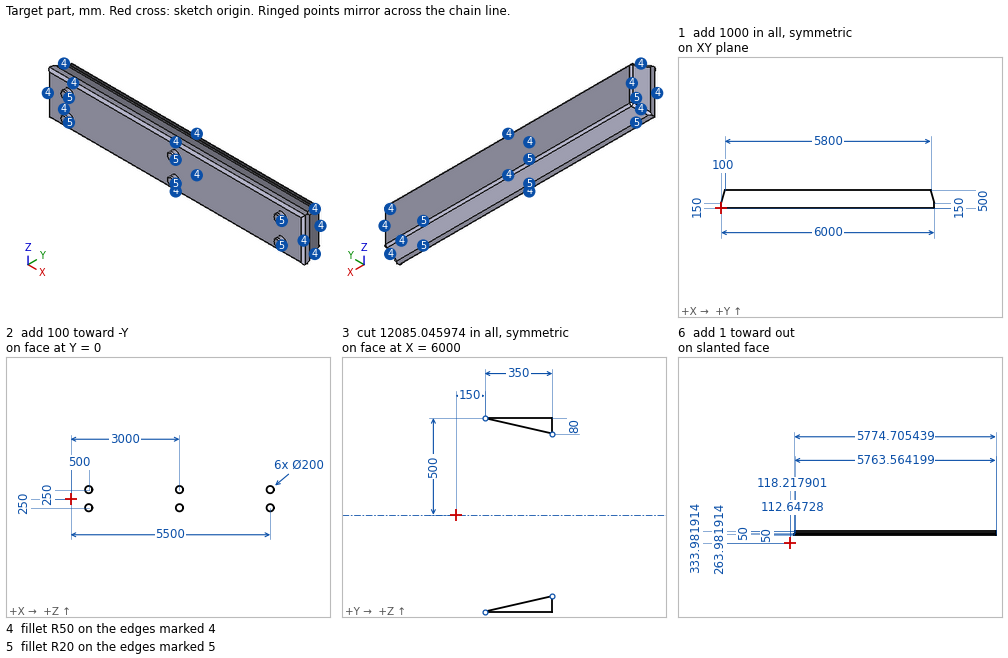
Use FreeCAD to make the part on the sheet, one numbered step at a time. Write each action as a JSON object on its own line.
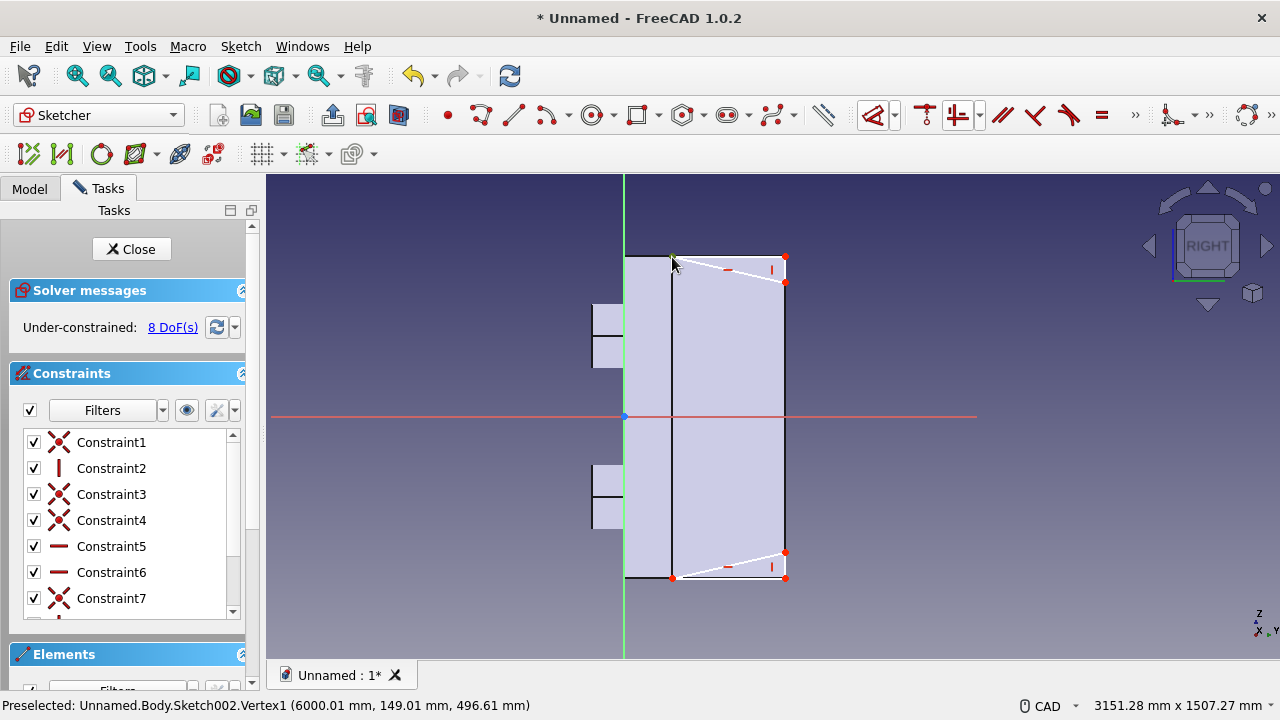
{"action": "left_click", "coordinate": [672, 579]}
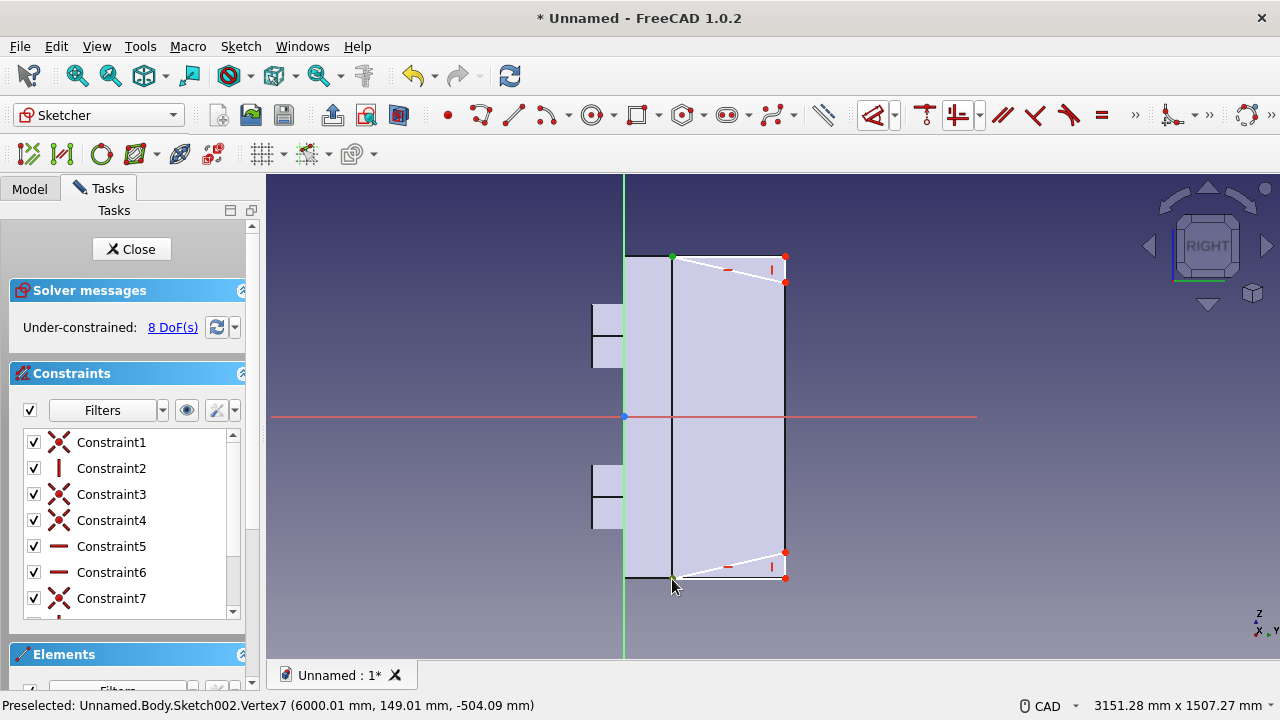
{"action": "left_click", "coordinate": [353, 417]}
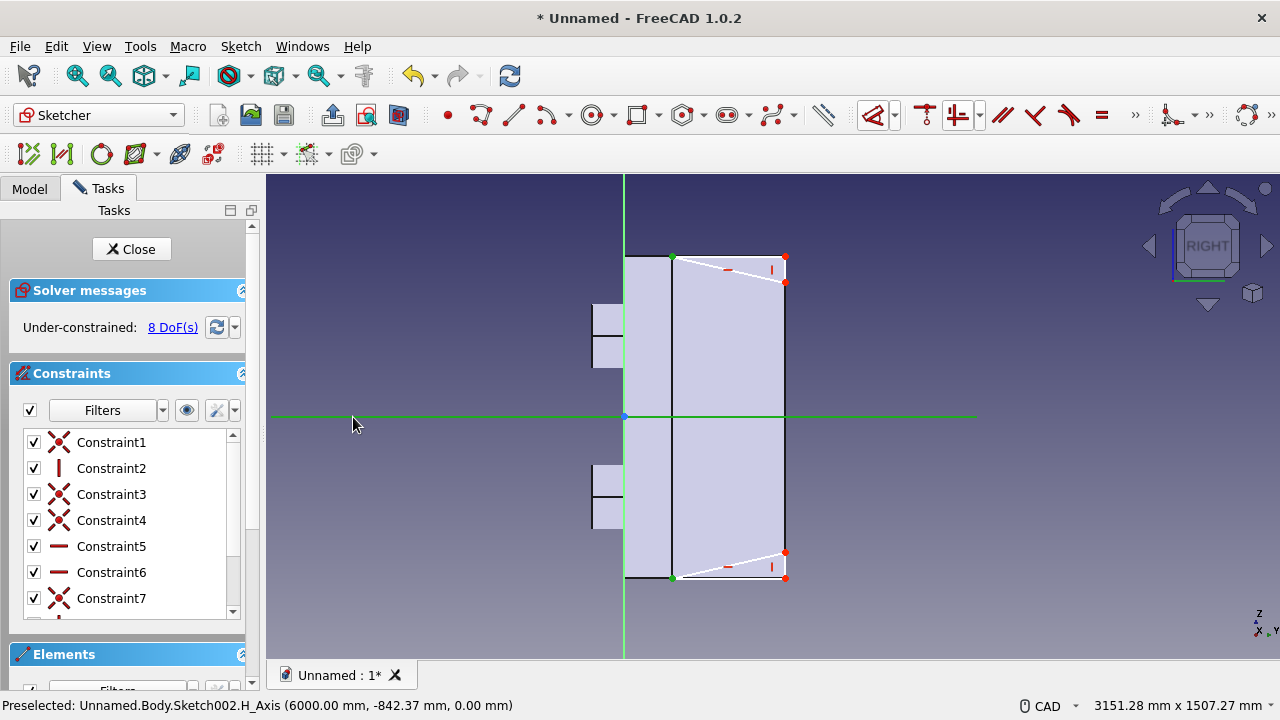
{"action": "key", "text": "s"}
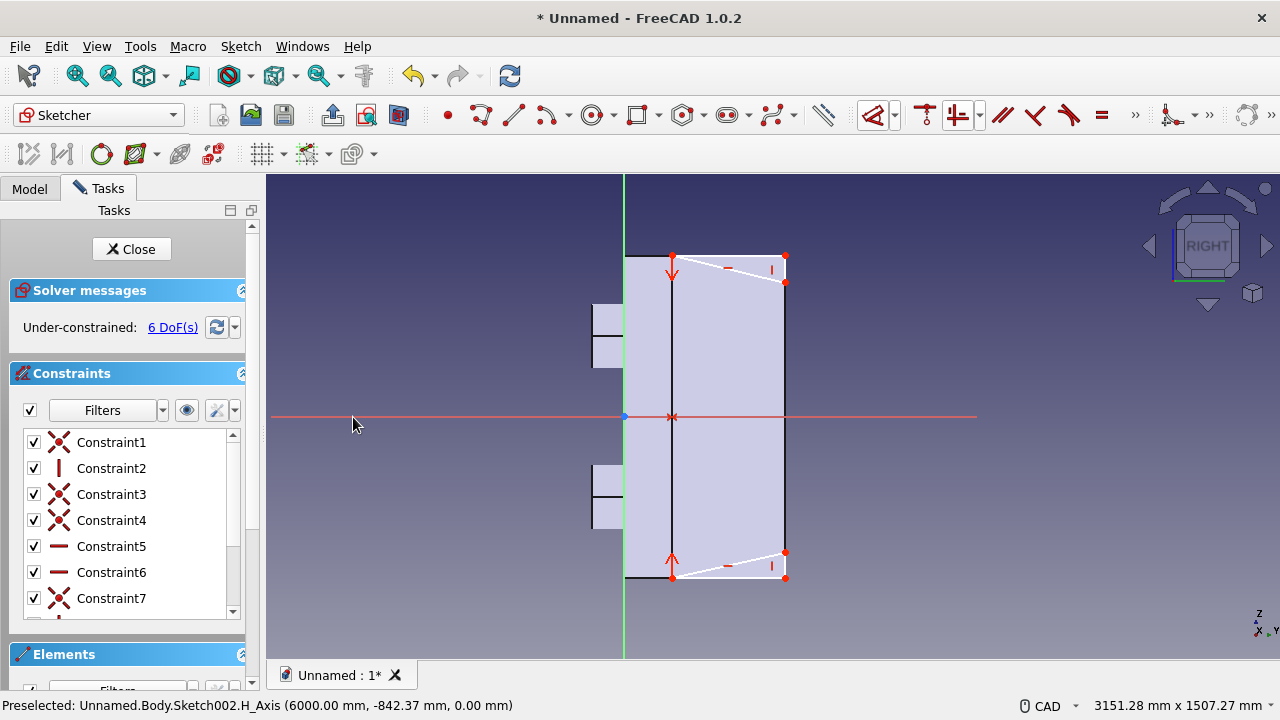
{"action": "left_click", "coordinate": [785, 283]}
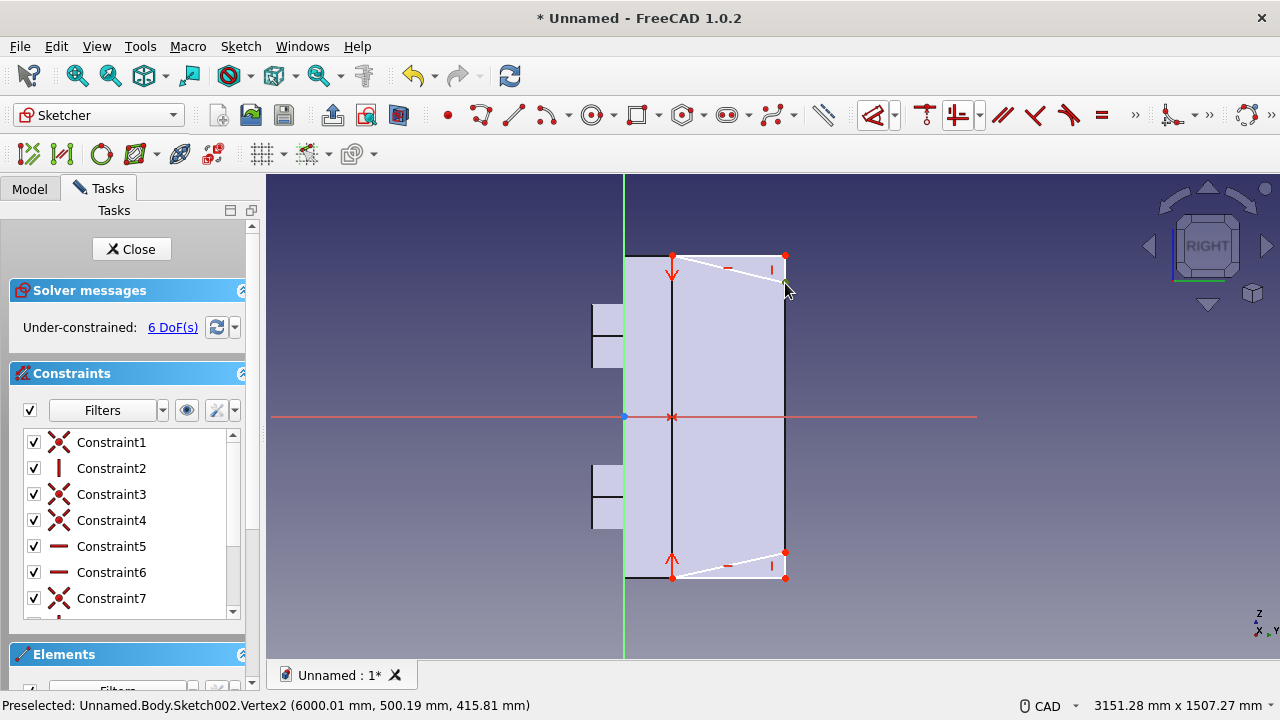
{"action": "left_click", "coordinate": [785, 553]}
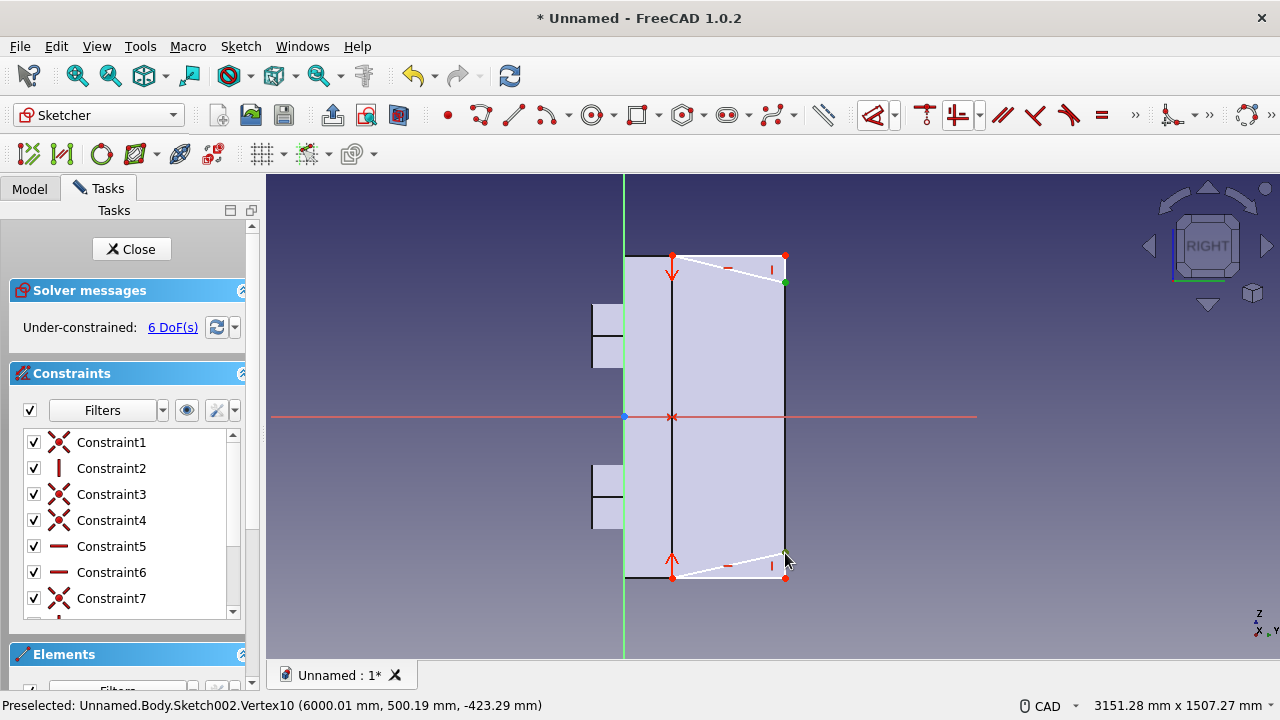
{"action": "left_click", "coordinate": [353, 417]}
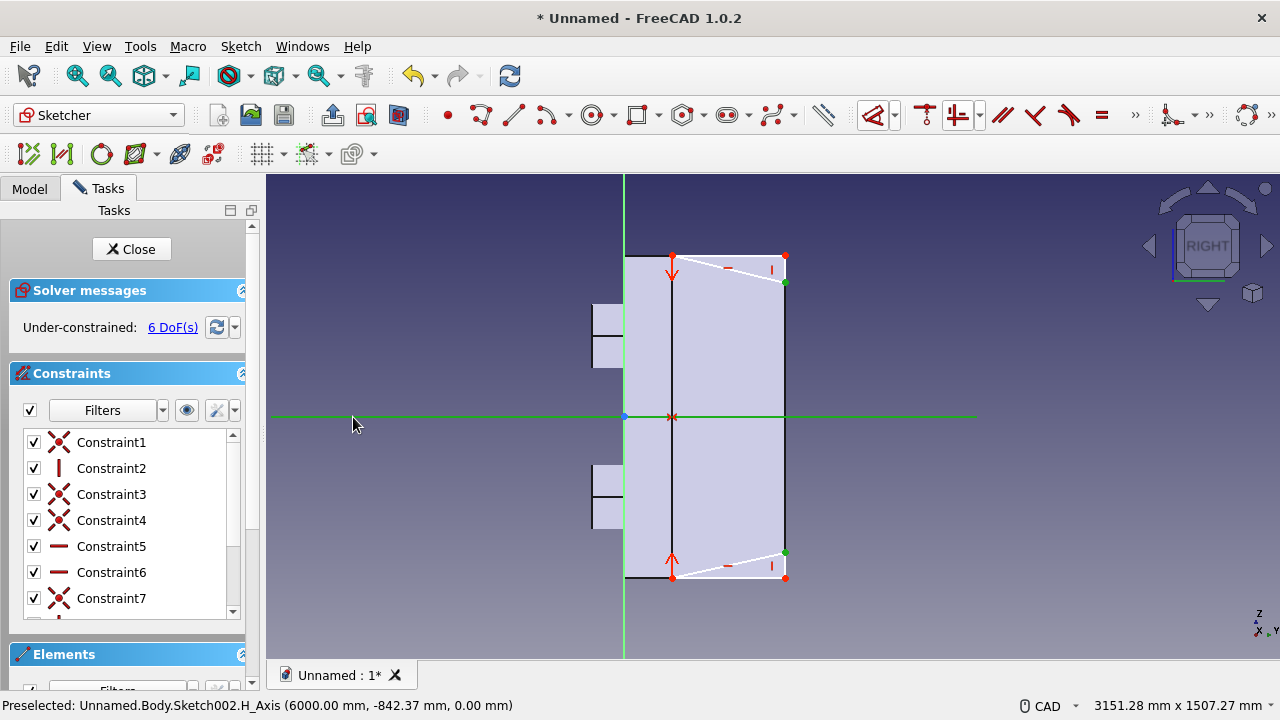
{"action": "key", "text": "s"}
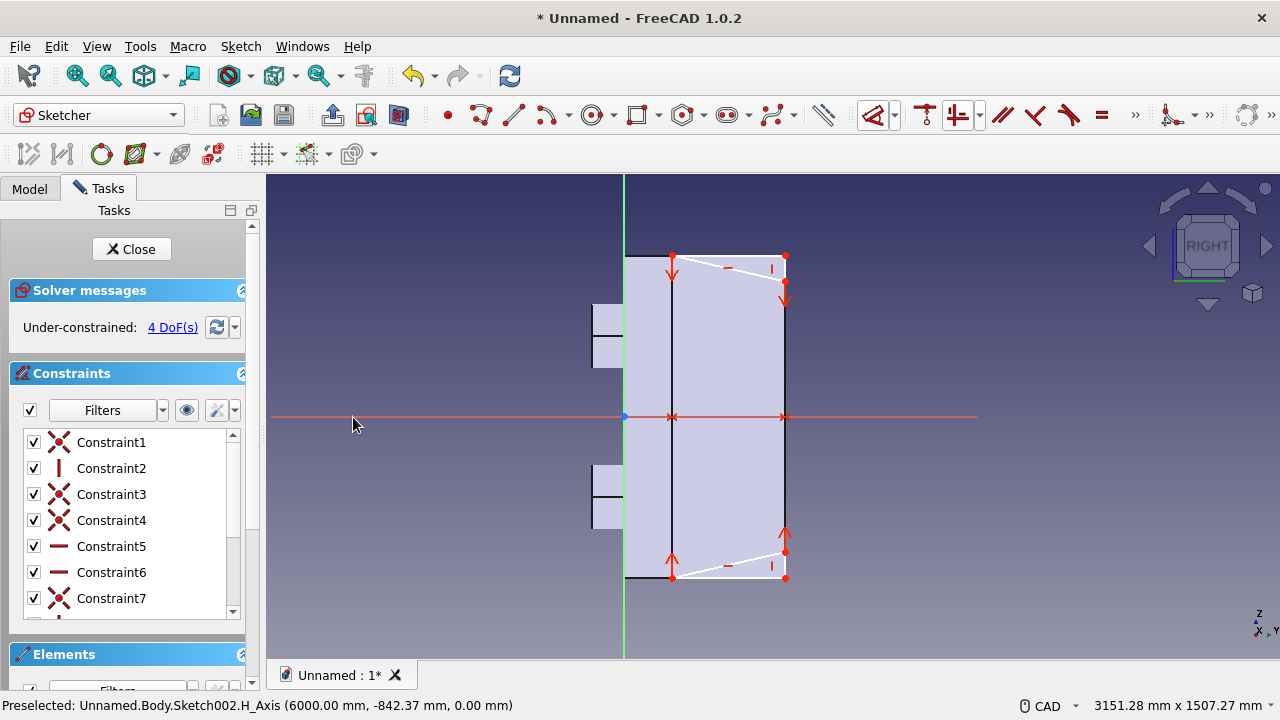
{"action": "scroll", "coordinate": [785, 271], "scroll_direction": "up", "scroll_amount": 3}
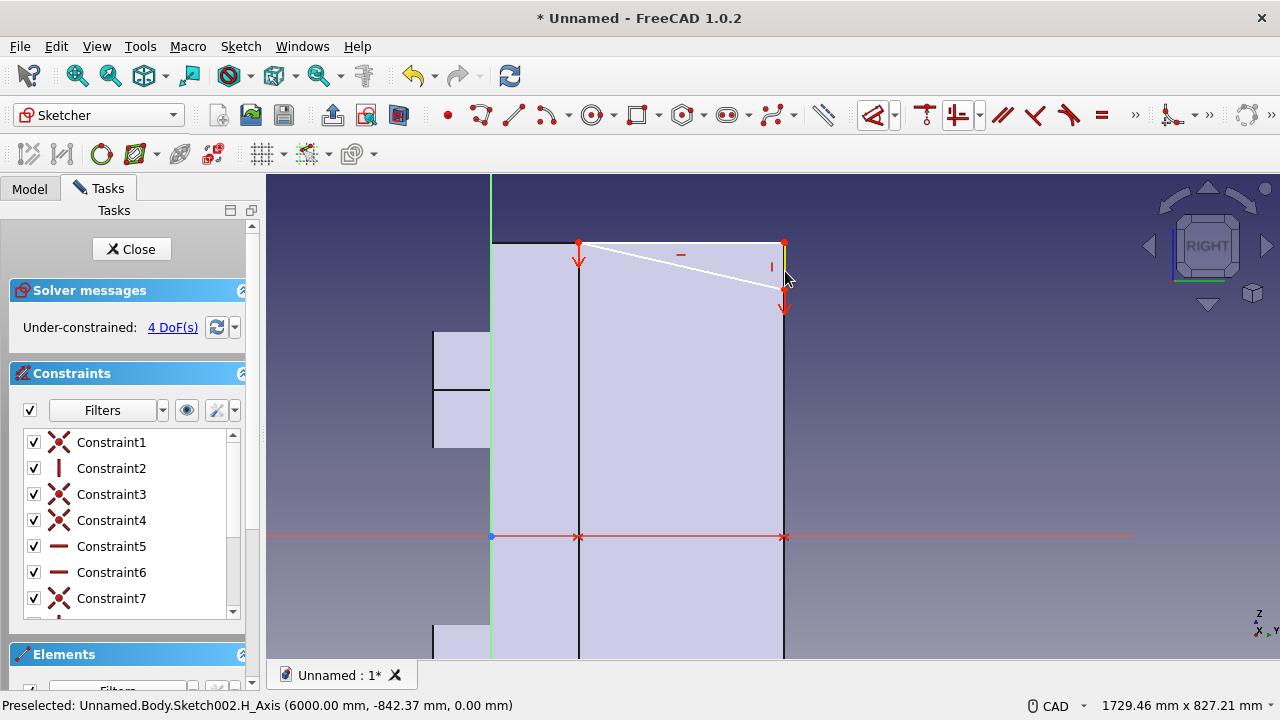
{"action": "left_click", "coordinate": [785, 271]}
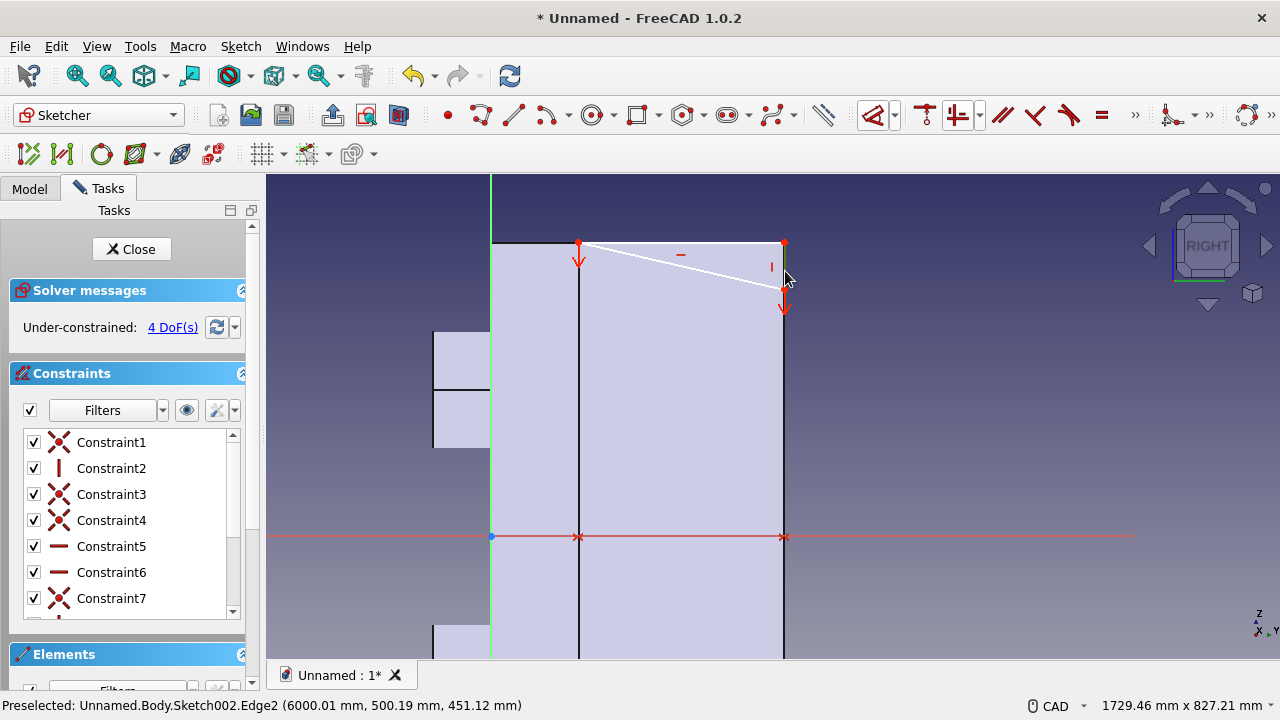
{"action": "left_click", "coordinate": [894, 116]}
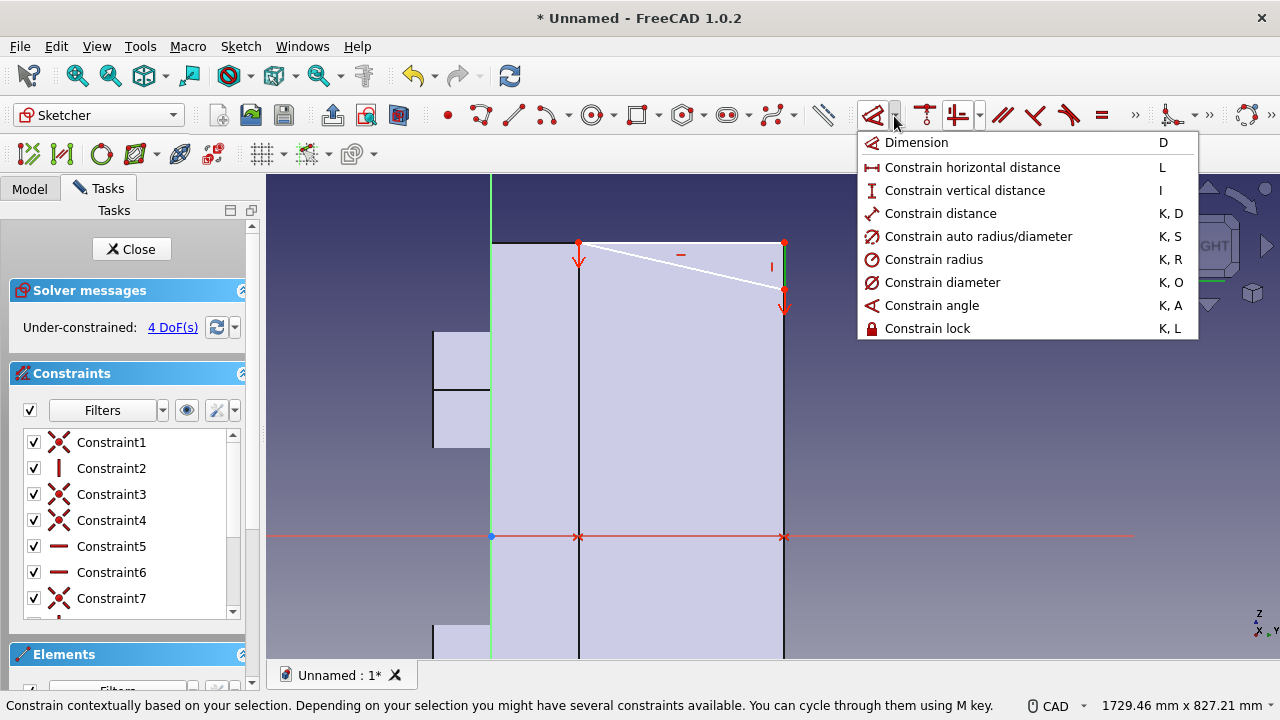
{"action": "left_click", "coordinate": [1028, 190]}